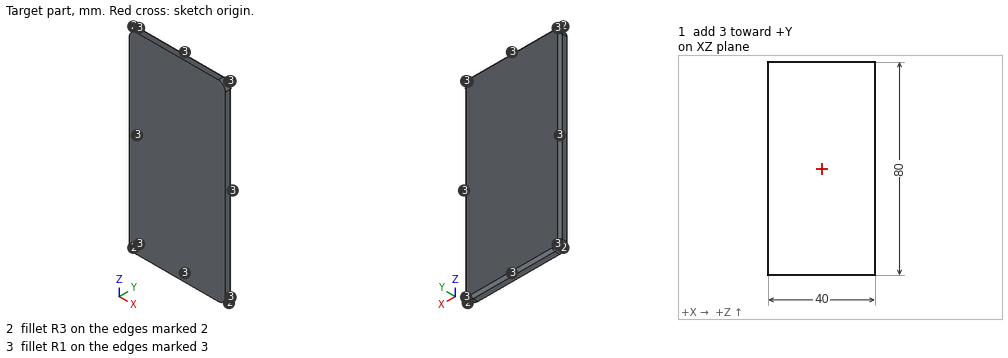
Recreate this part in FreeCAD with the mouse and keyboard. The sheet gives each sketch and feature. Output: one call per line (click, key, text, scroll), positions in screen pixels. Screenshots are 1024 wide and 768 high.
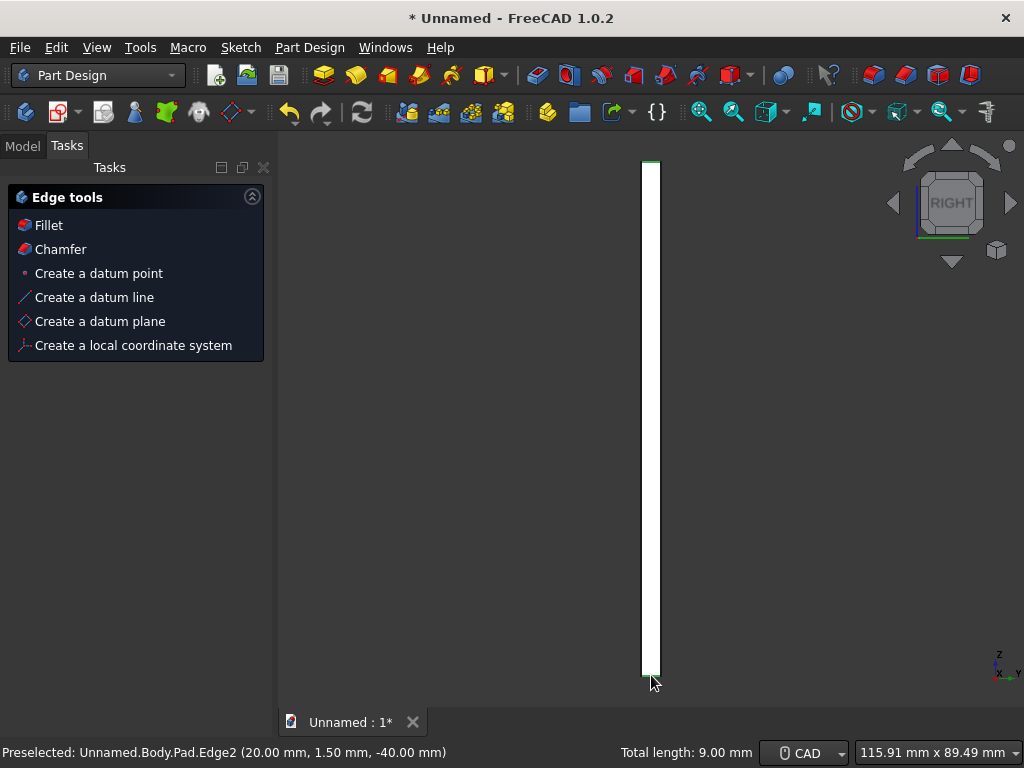
scroll(651, 675, up, 4)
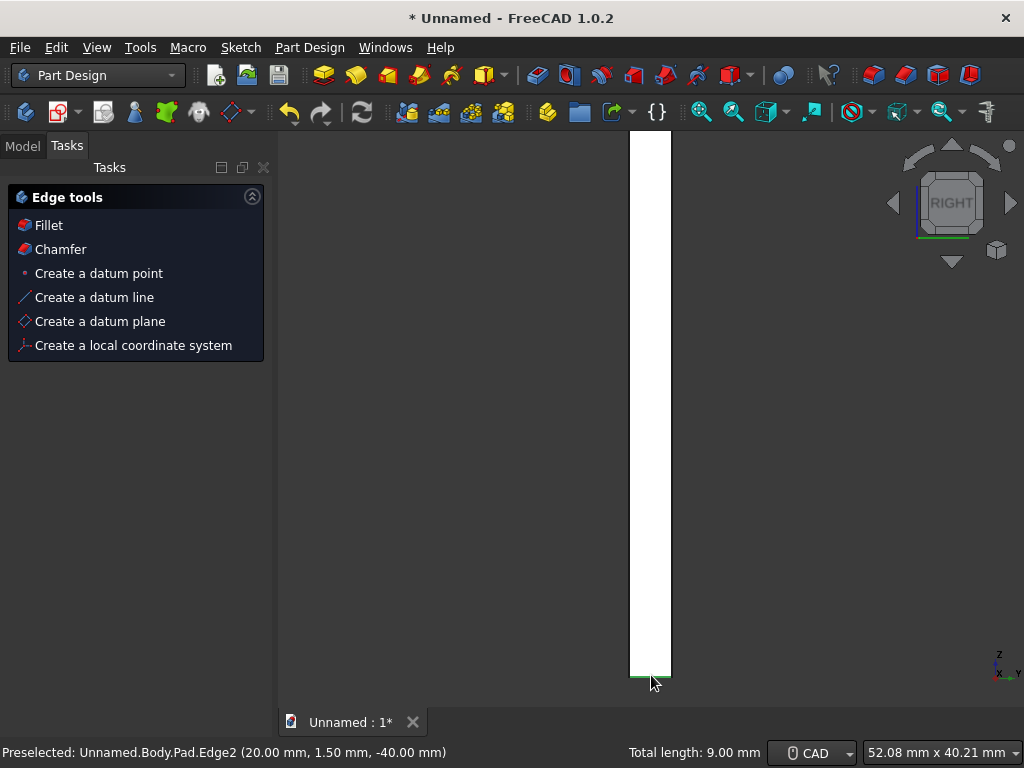
key(v)
key(f)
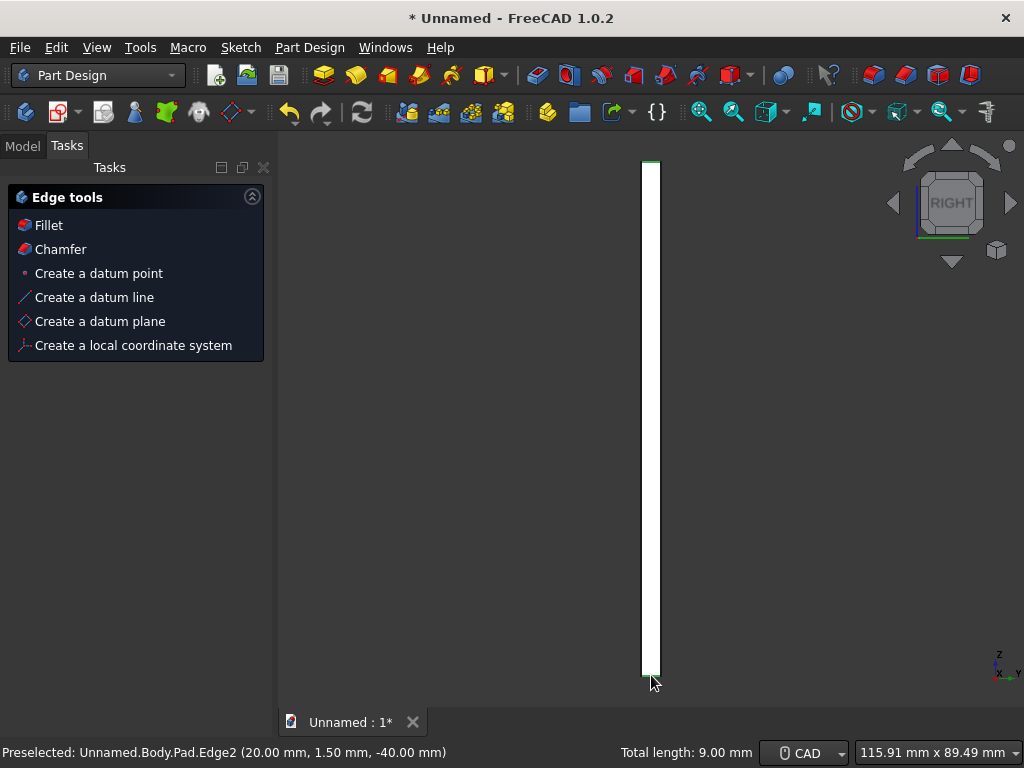
key(5)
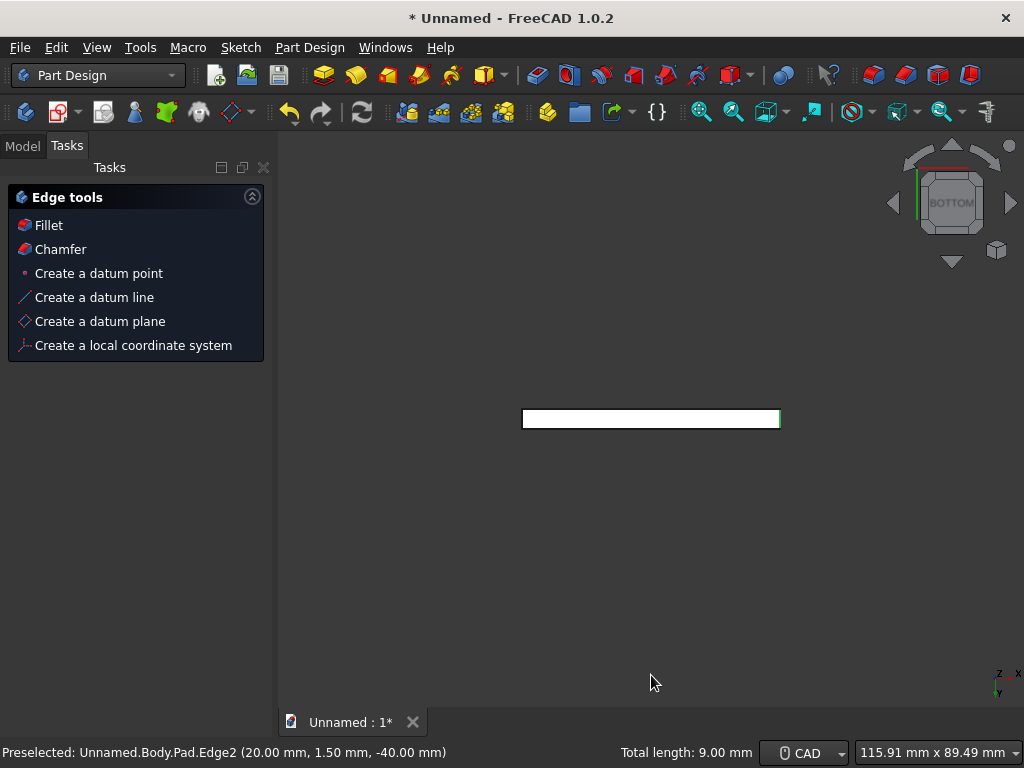
key(v)
key(f)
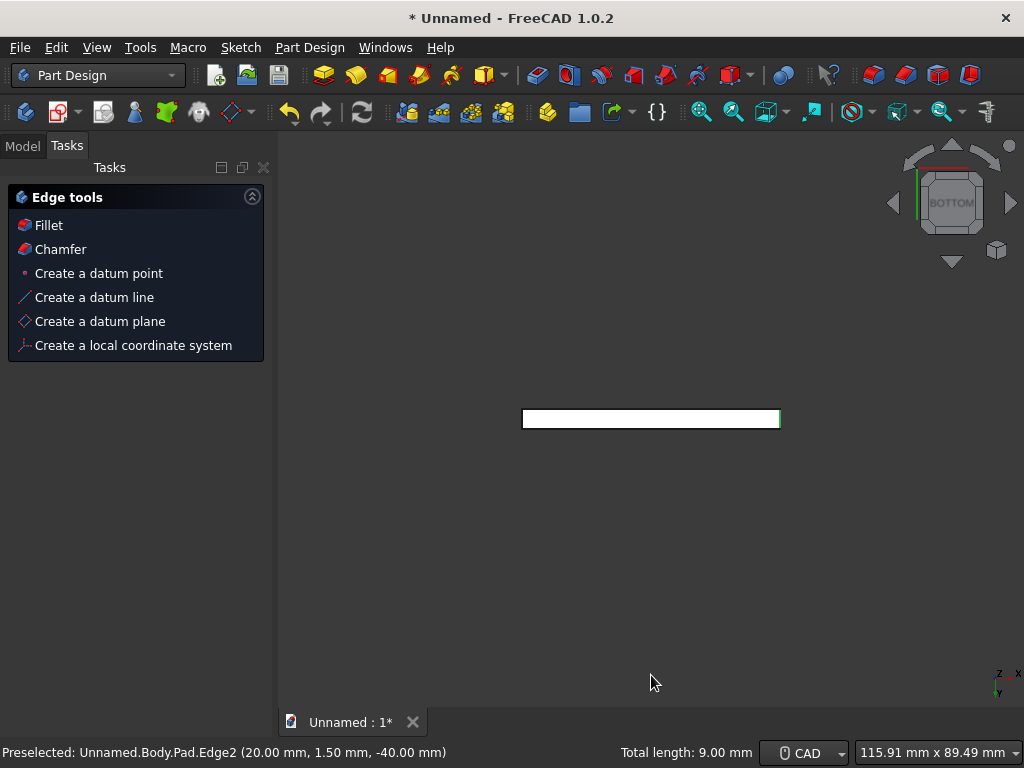
click(522, 418, ctrl)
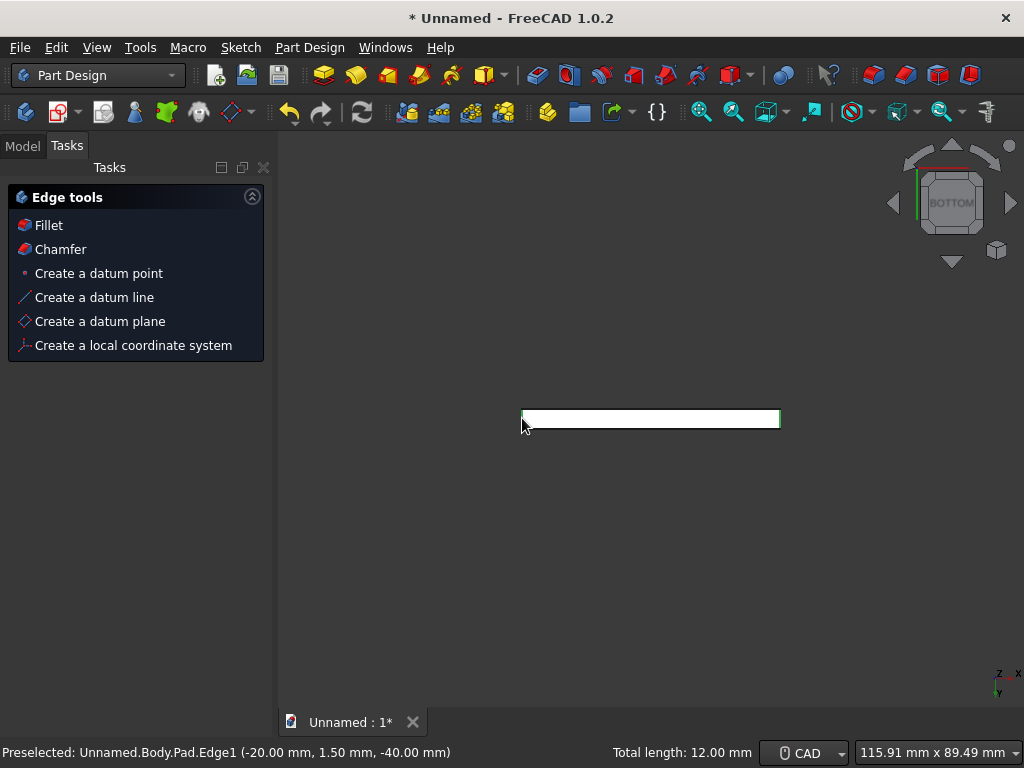
click(874, 76)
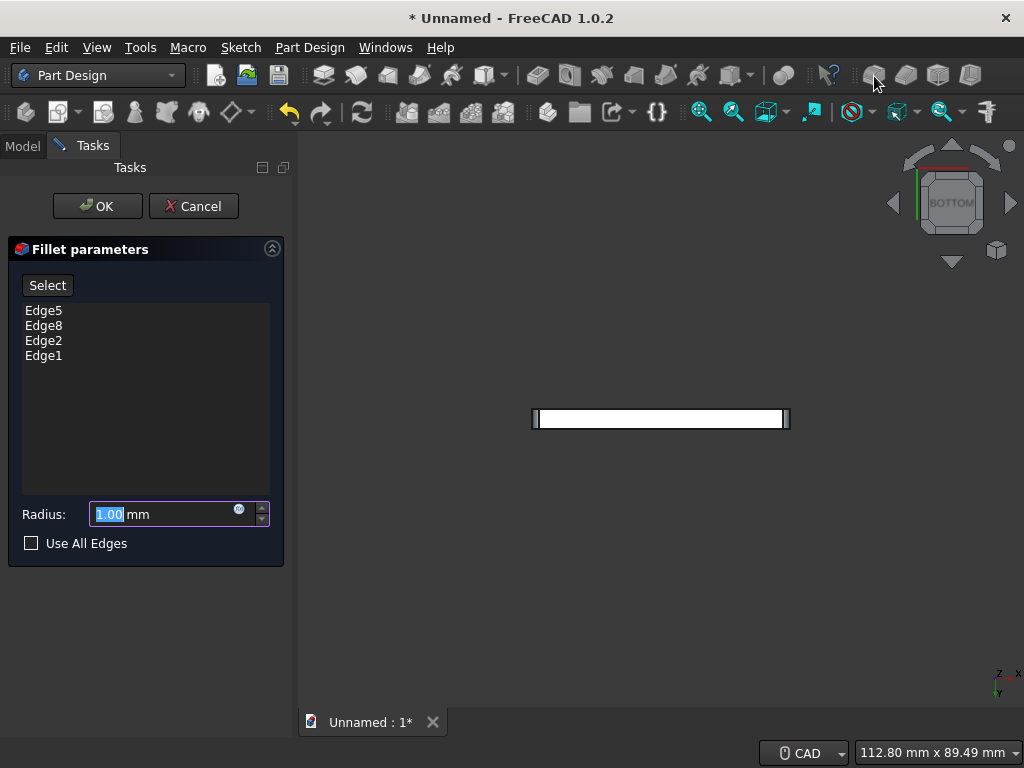
text(3)
key(Tab)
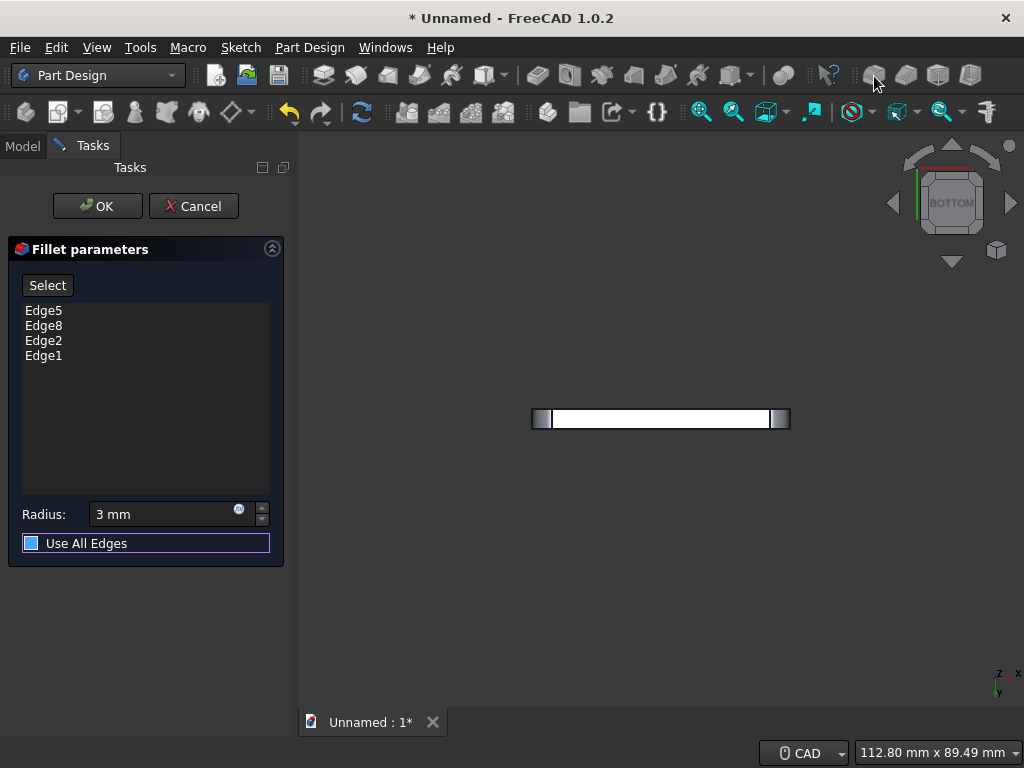
click(98, 206)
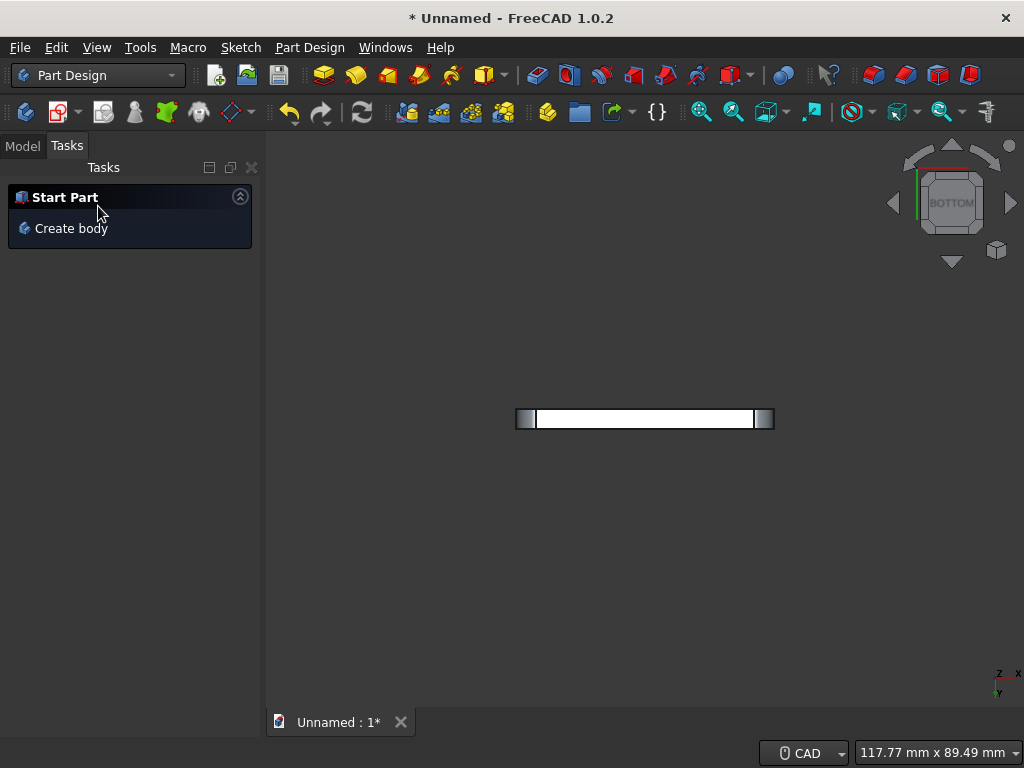
click(702, 112)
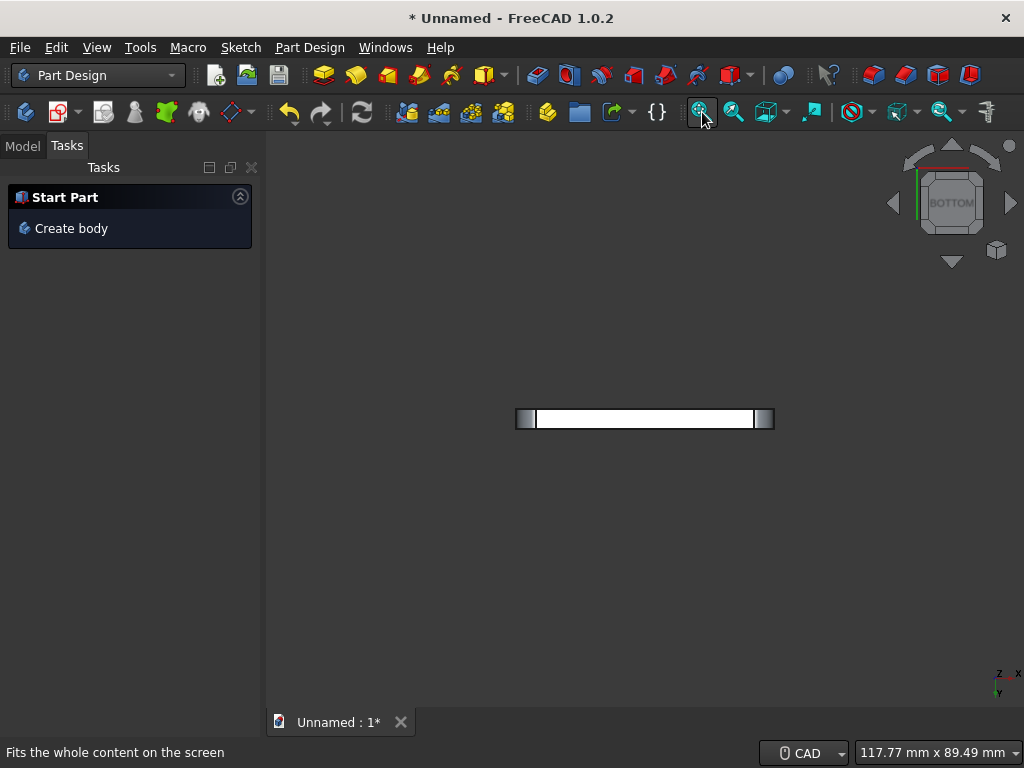
key(0)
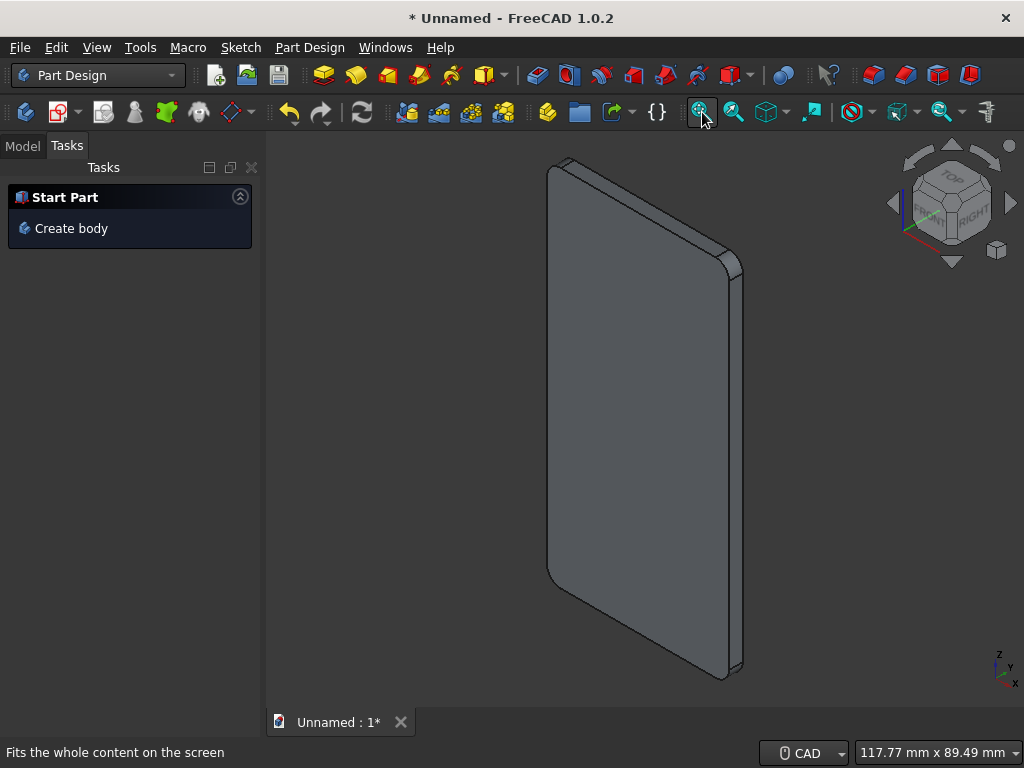
key(2)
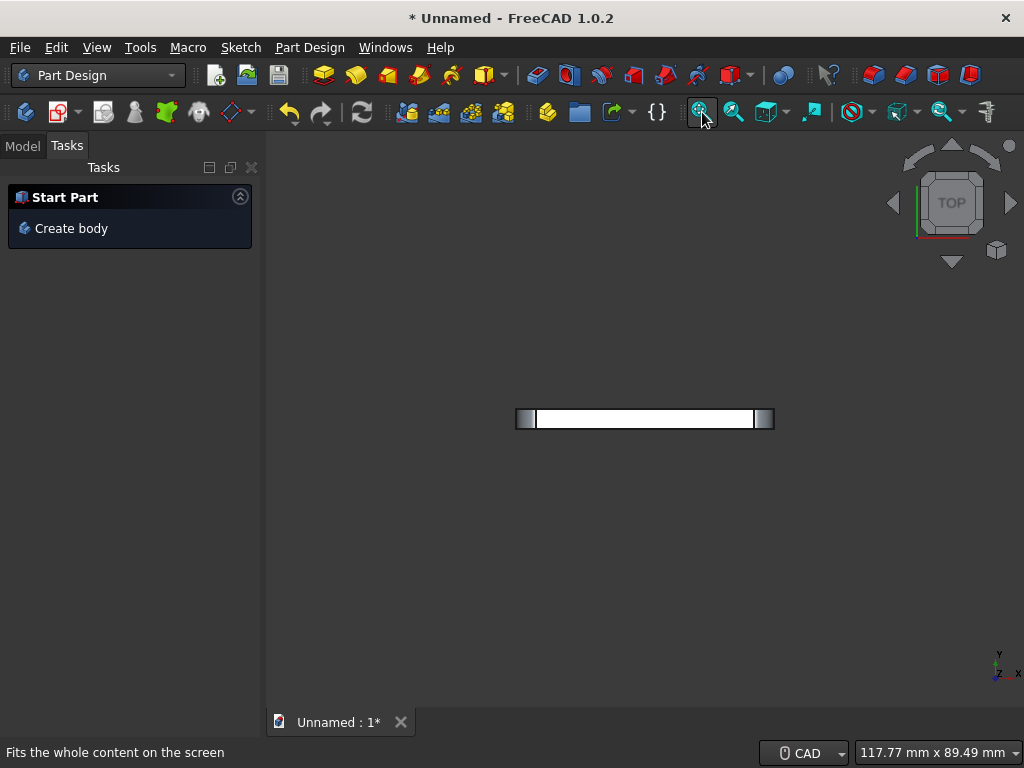
click(702, 112)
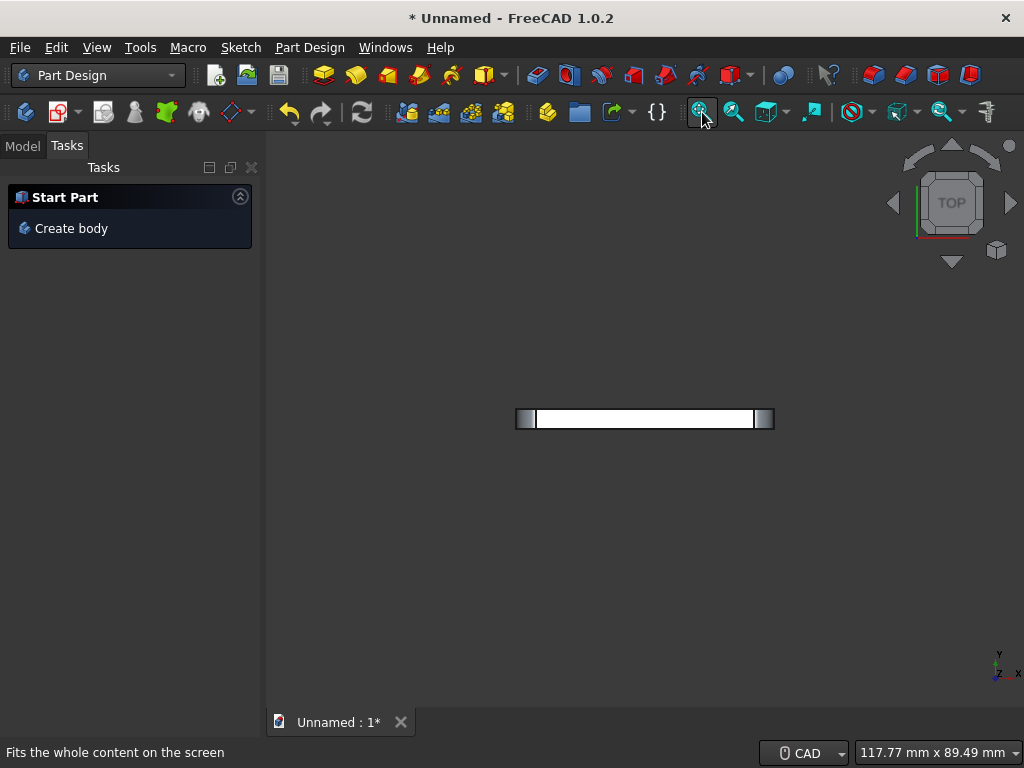
key(1)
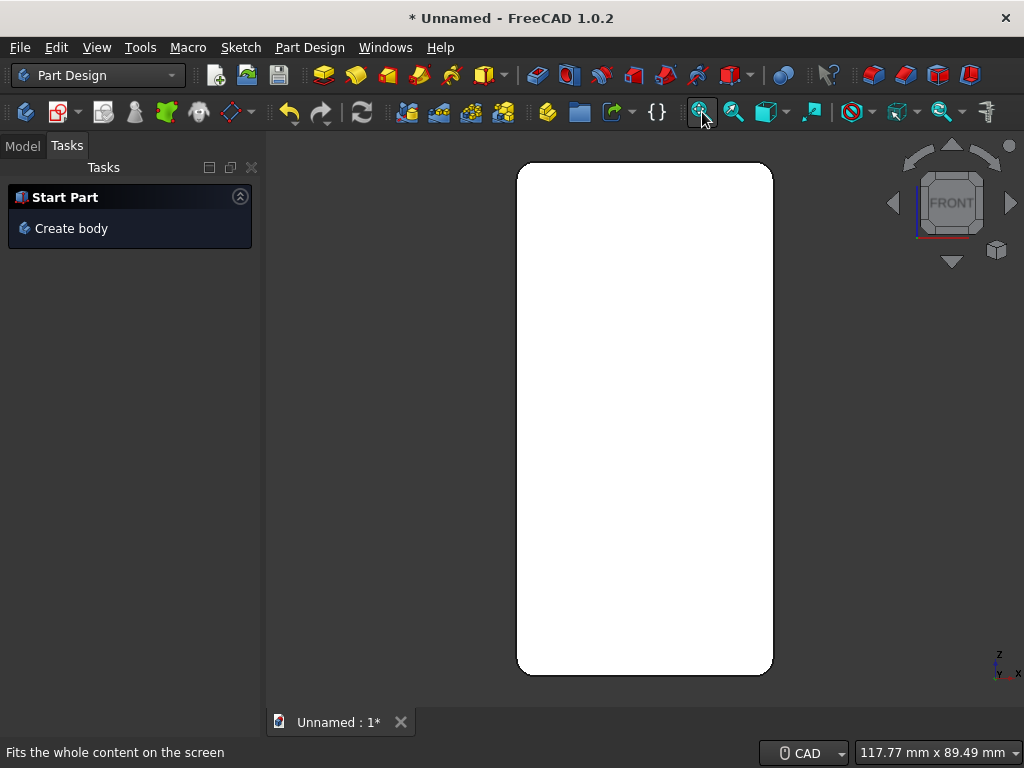
key(3)